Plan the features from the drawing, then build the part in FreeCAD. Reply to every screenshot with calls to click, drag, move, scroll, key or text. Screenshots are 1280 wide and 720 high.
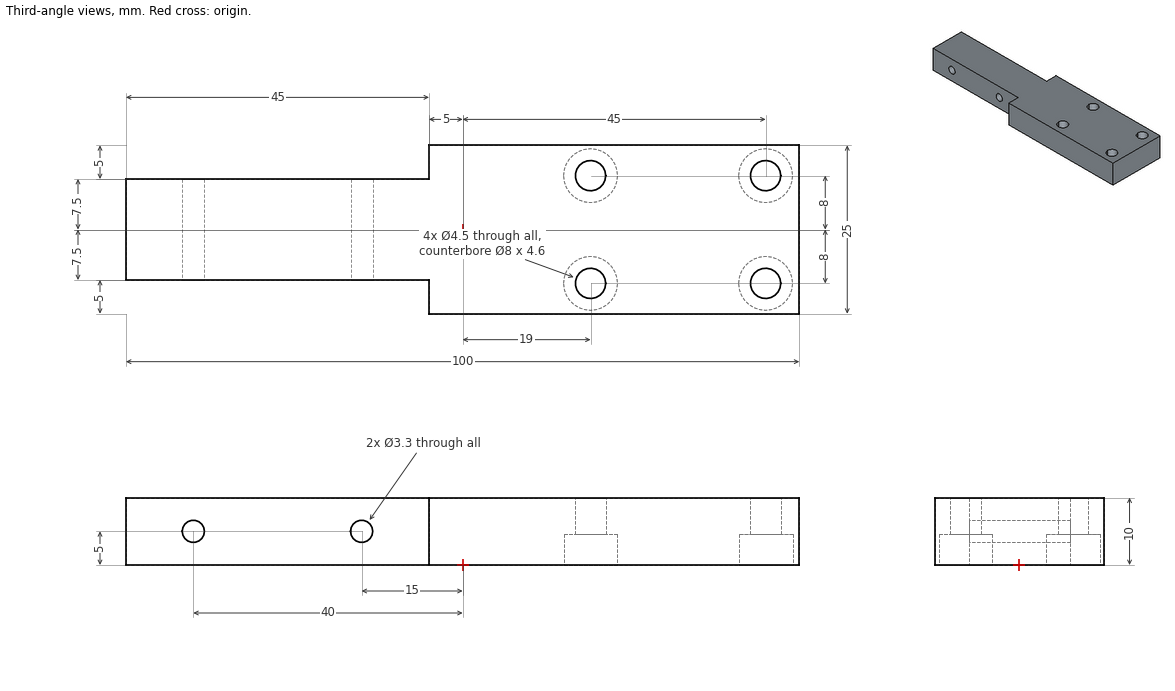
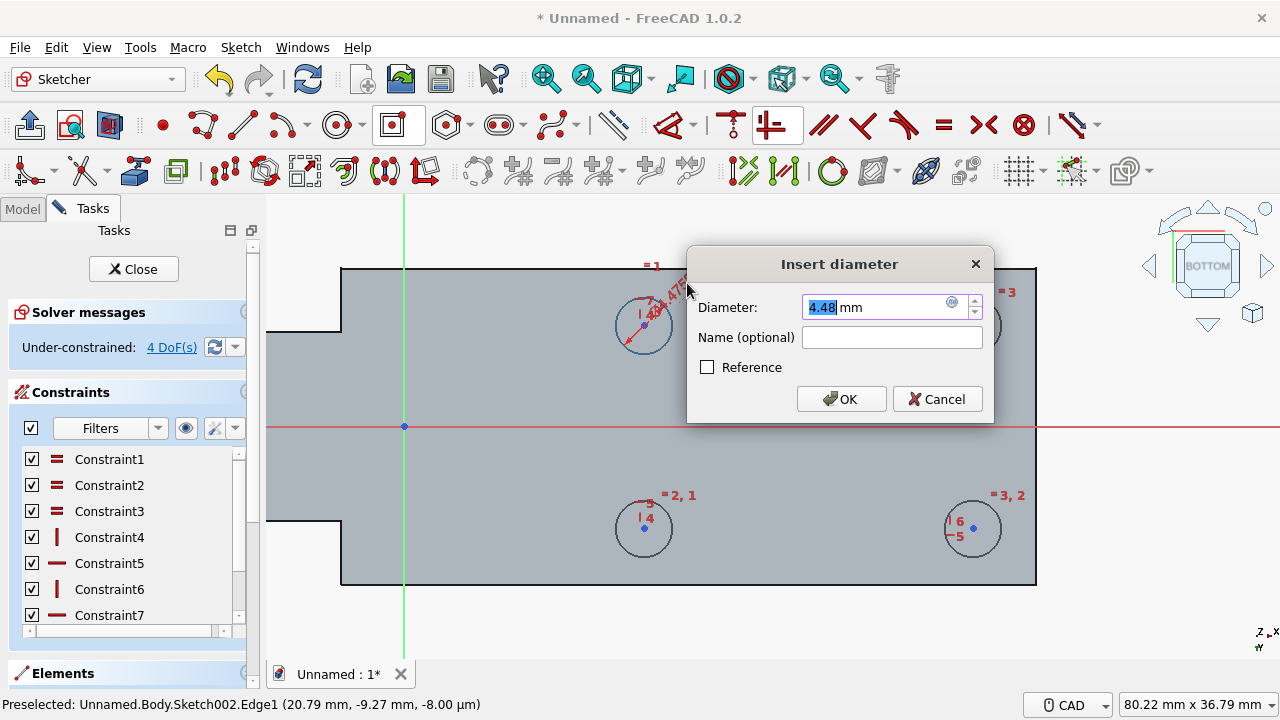
text(4.5)
key(Return)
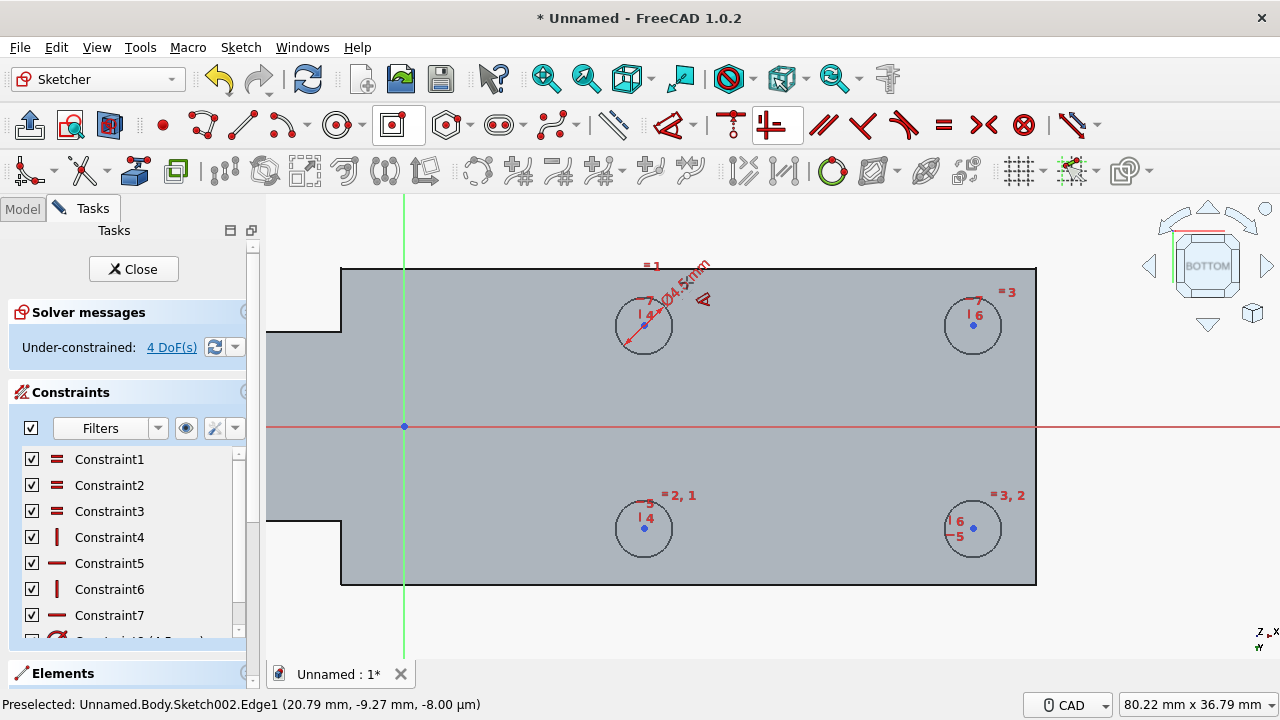
click(644, 326)
click(370, 376)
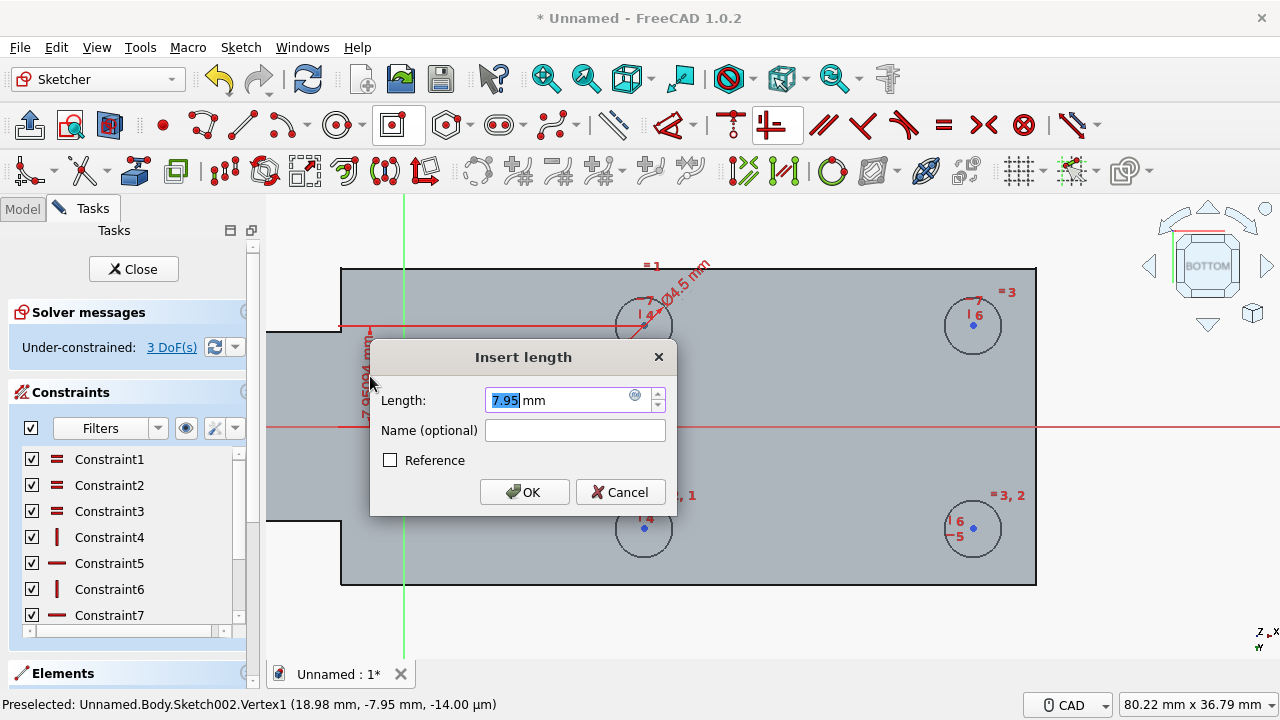
text(8)
key(Return)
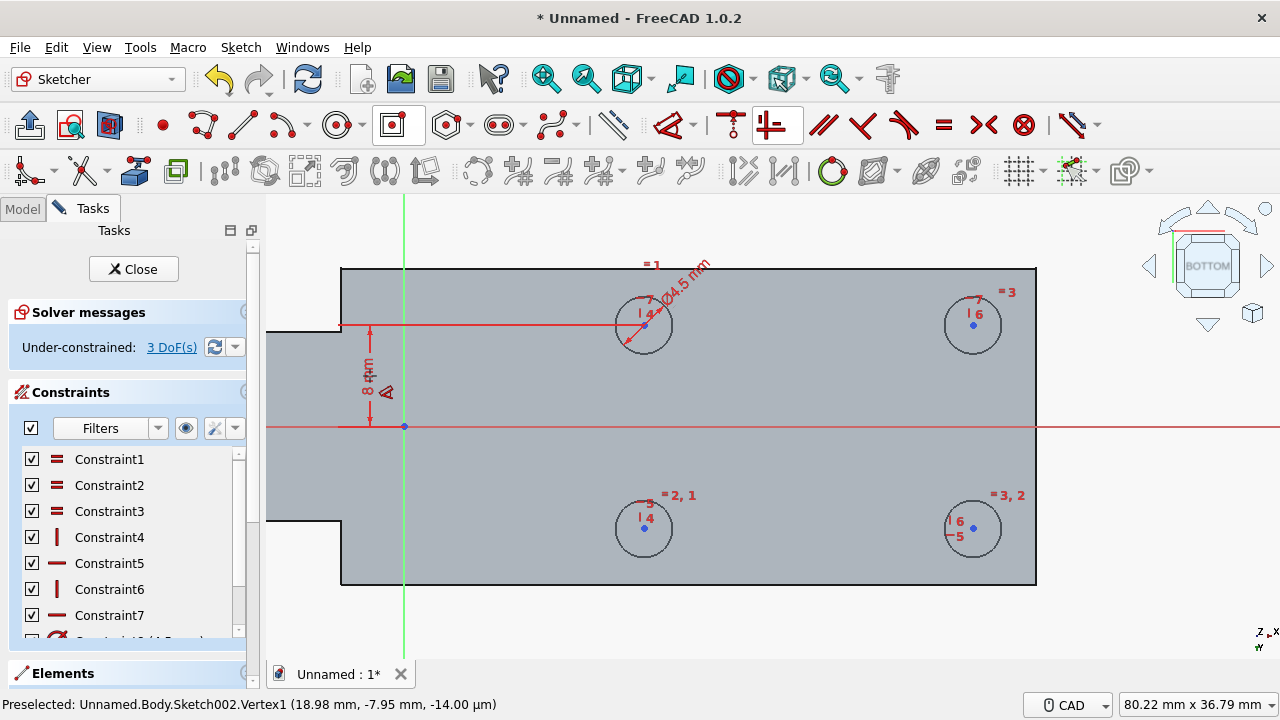
click(644, 529)
click(370, 478)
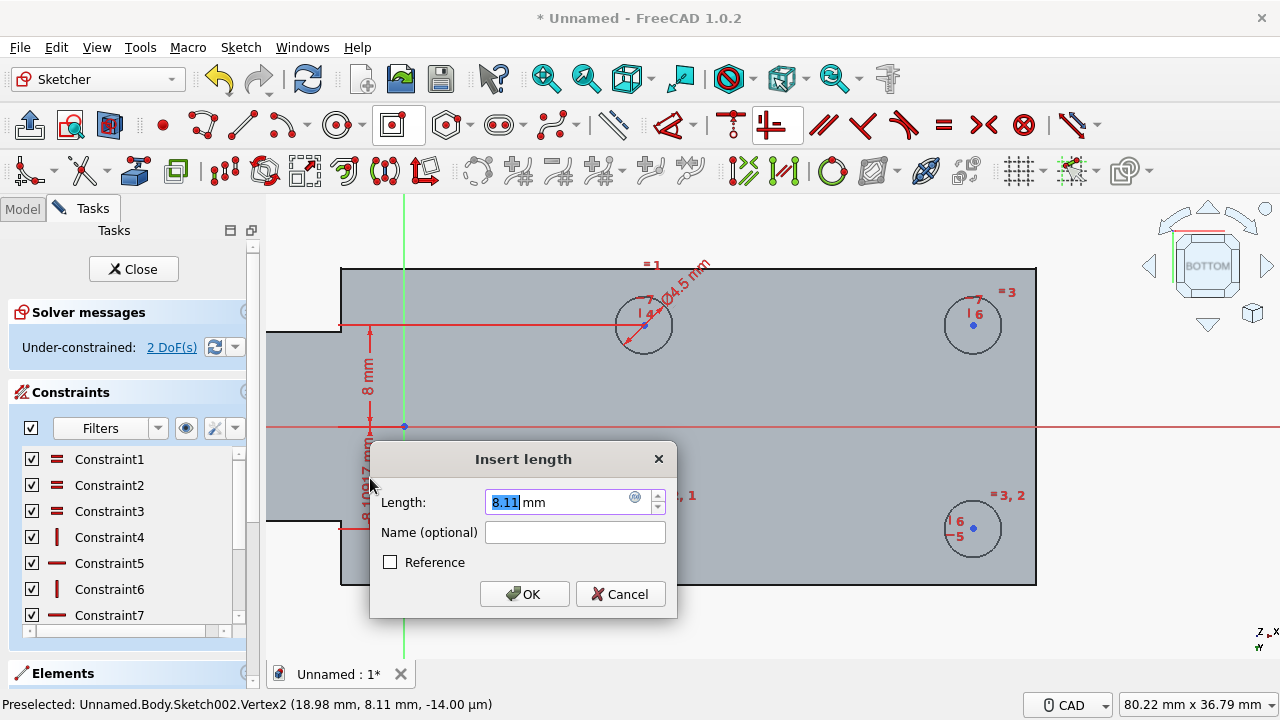
text(8)
key(Return)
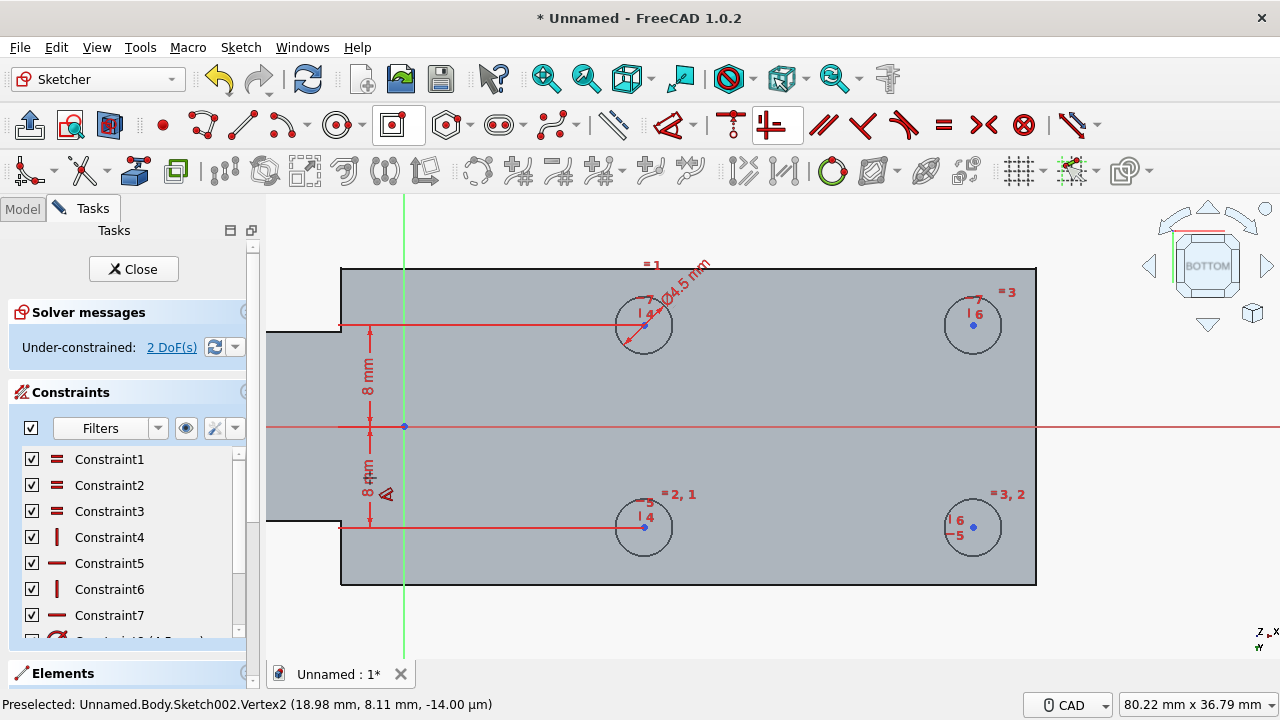
click(644, 325)
click(524, 291)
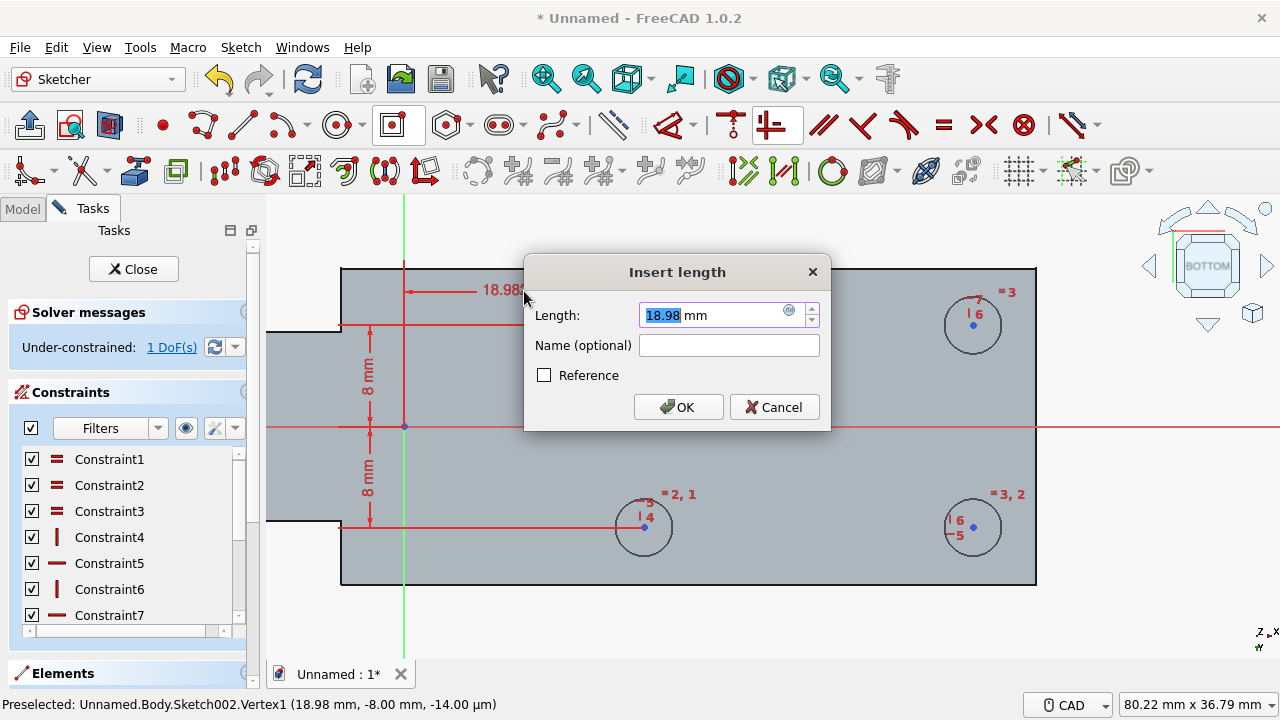
text(19)
key(Return)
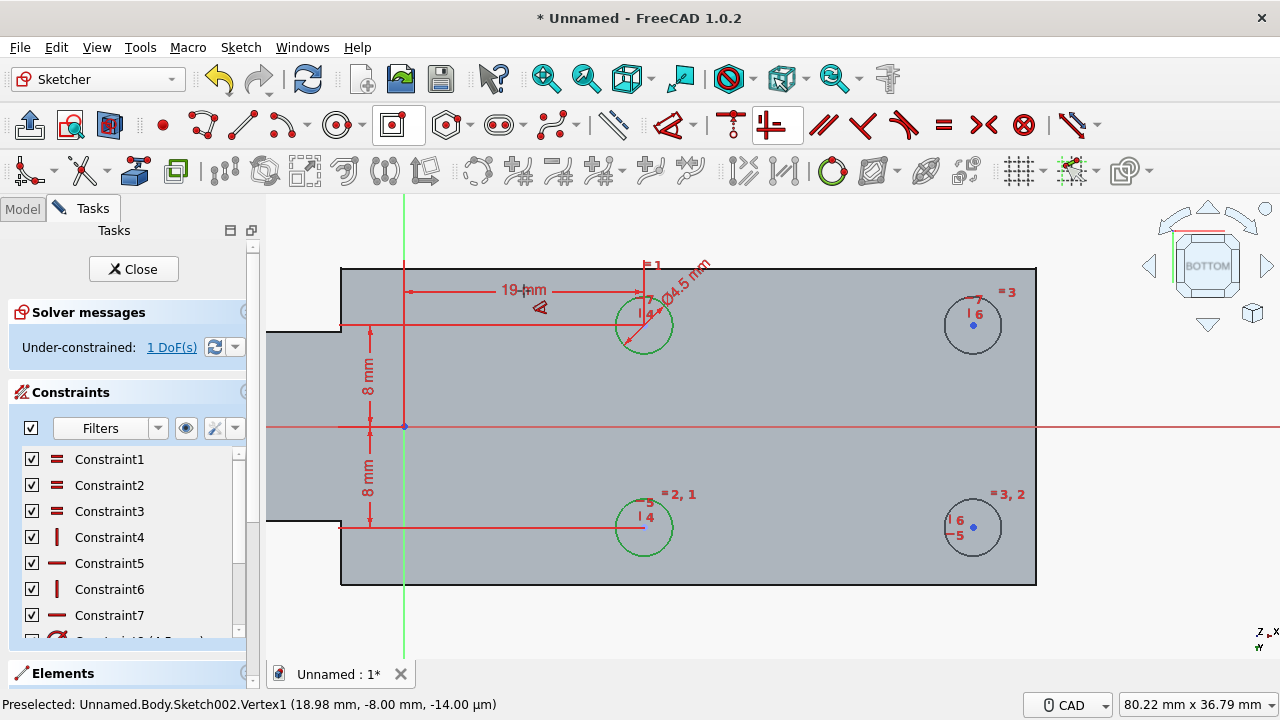
click(973, 528)
click(689, 562)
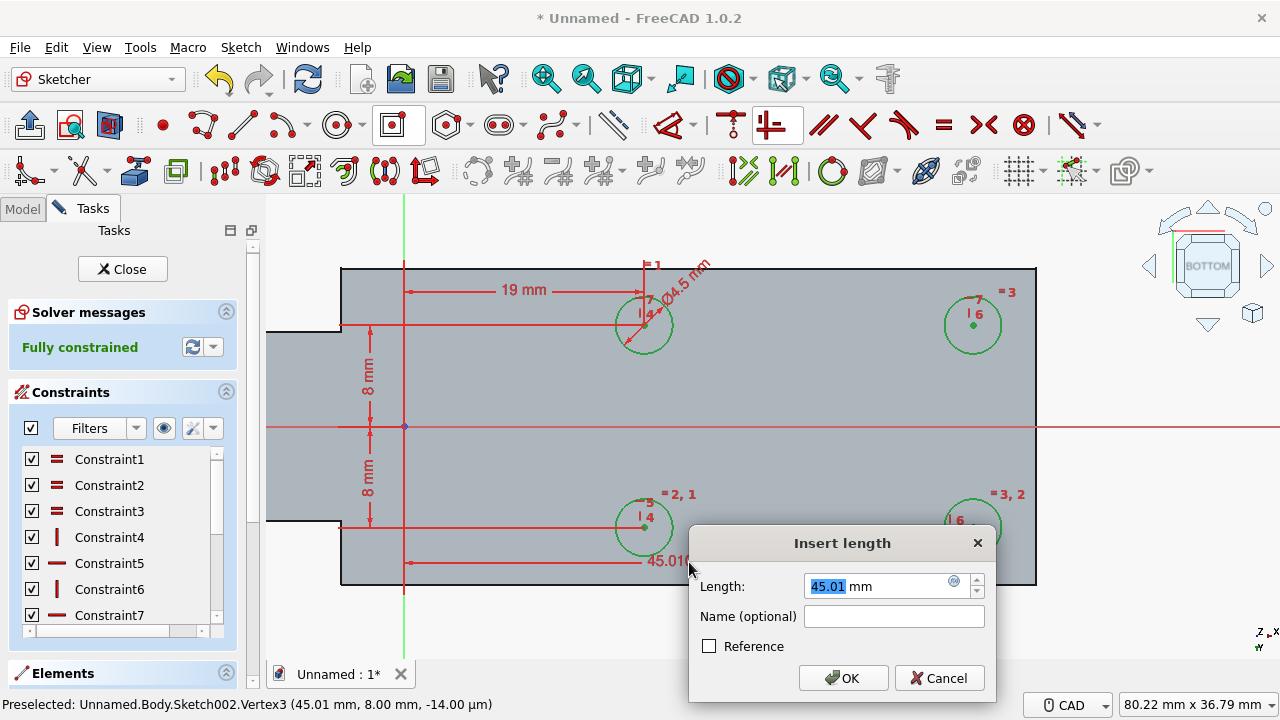
text(45)
key(Return)
key(Escape)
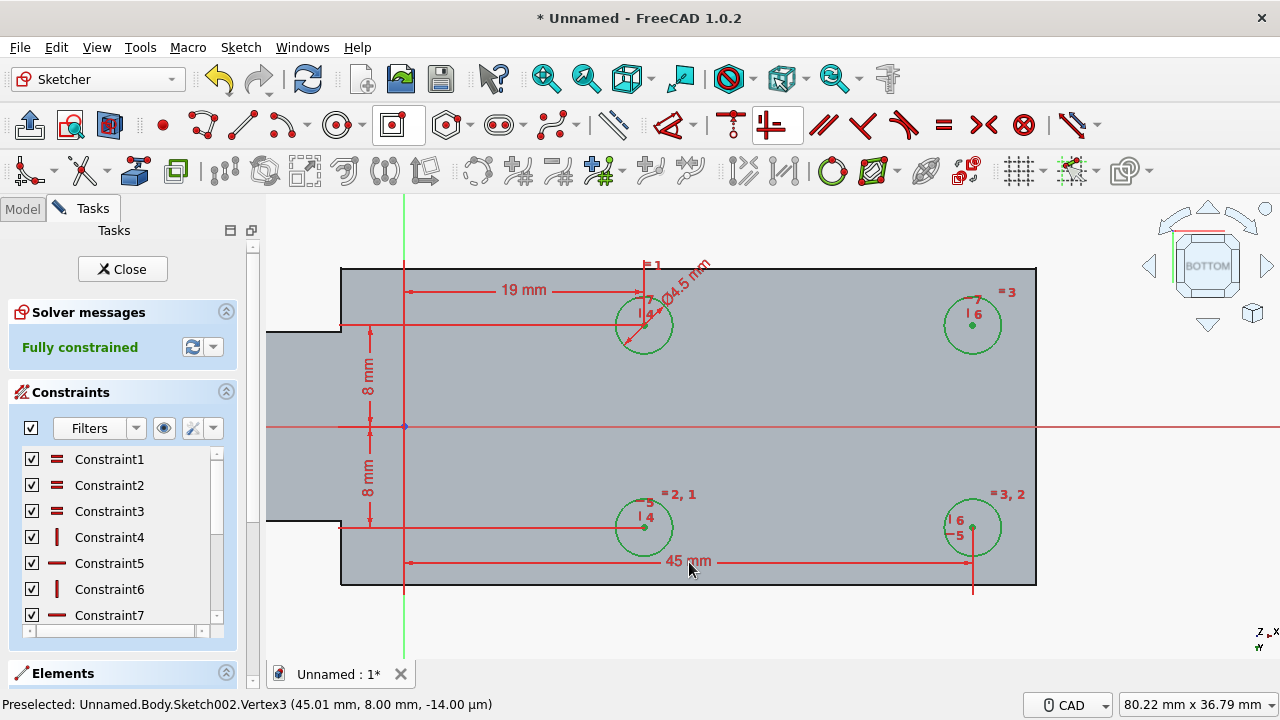
click(123, 269)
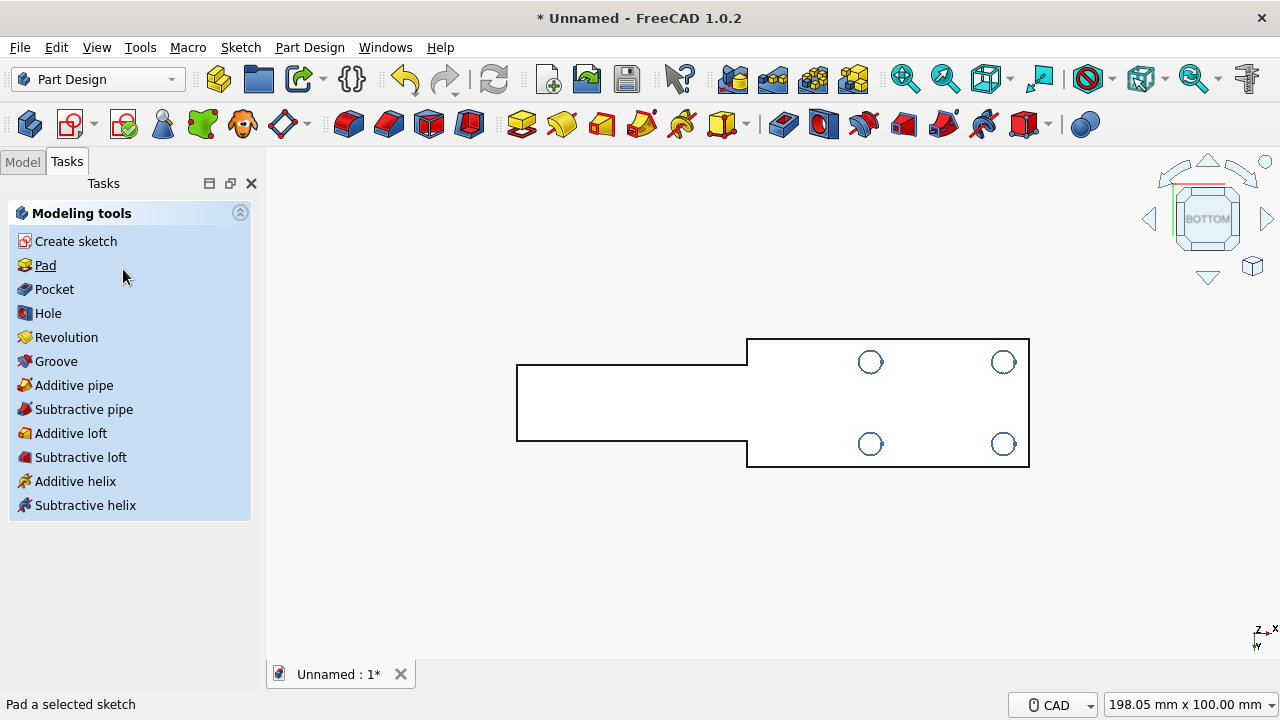
click(824, 124)